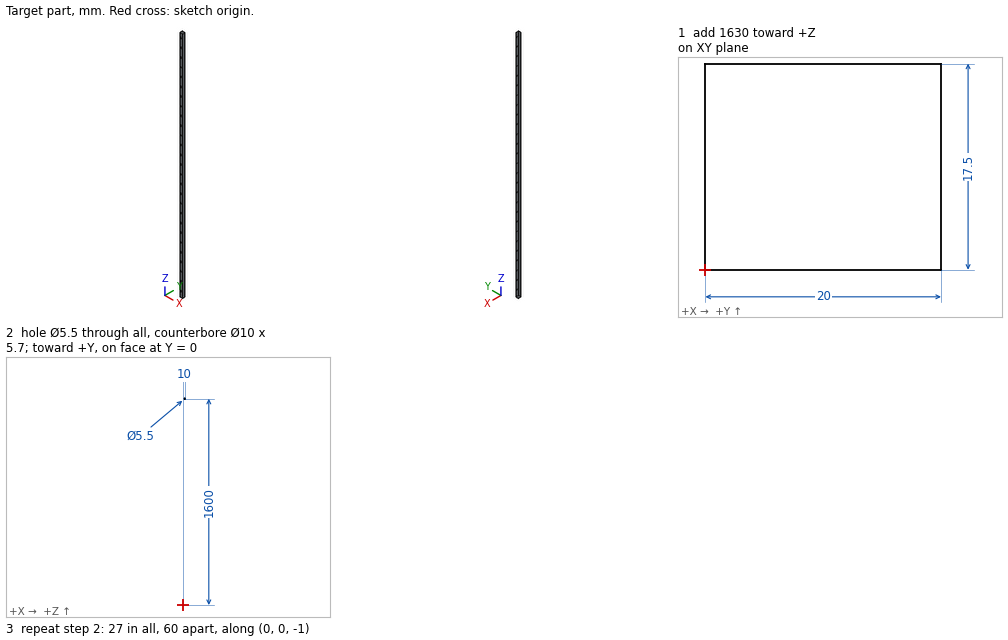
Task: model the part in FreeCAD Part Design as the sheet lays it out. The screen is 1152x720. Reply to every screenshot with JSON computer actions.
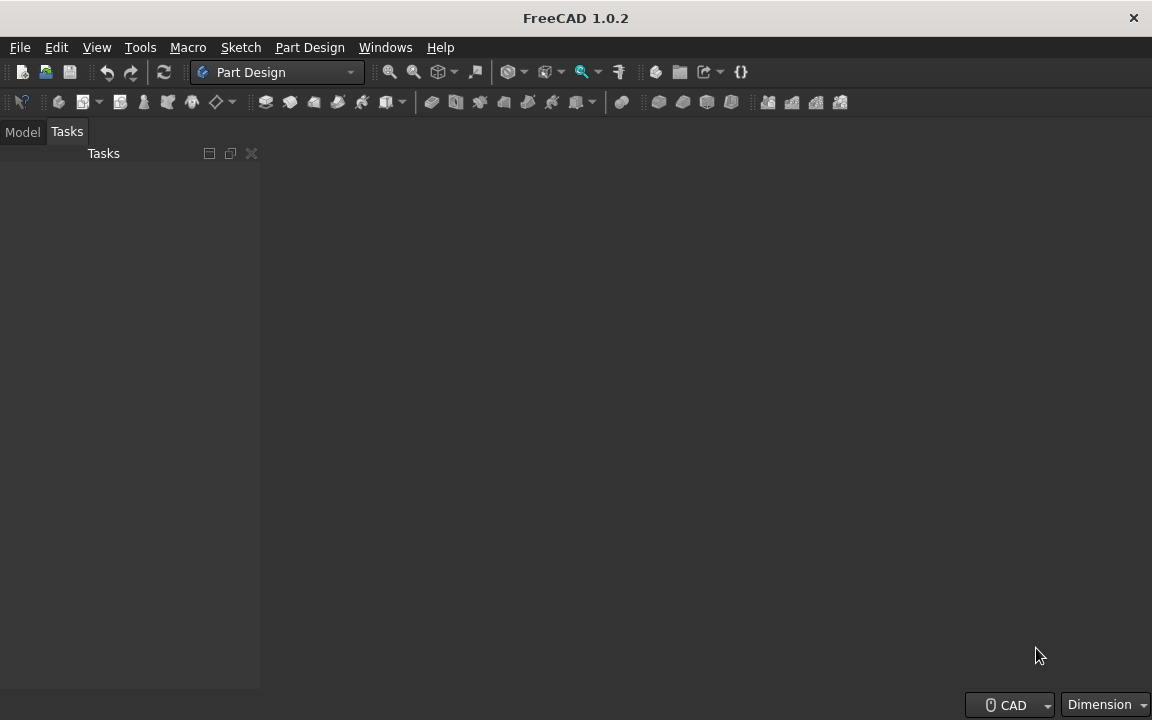
{"action": "left_click", "coordinate": [22, 72]}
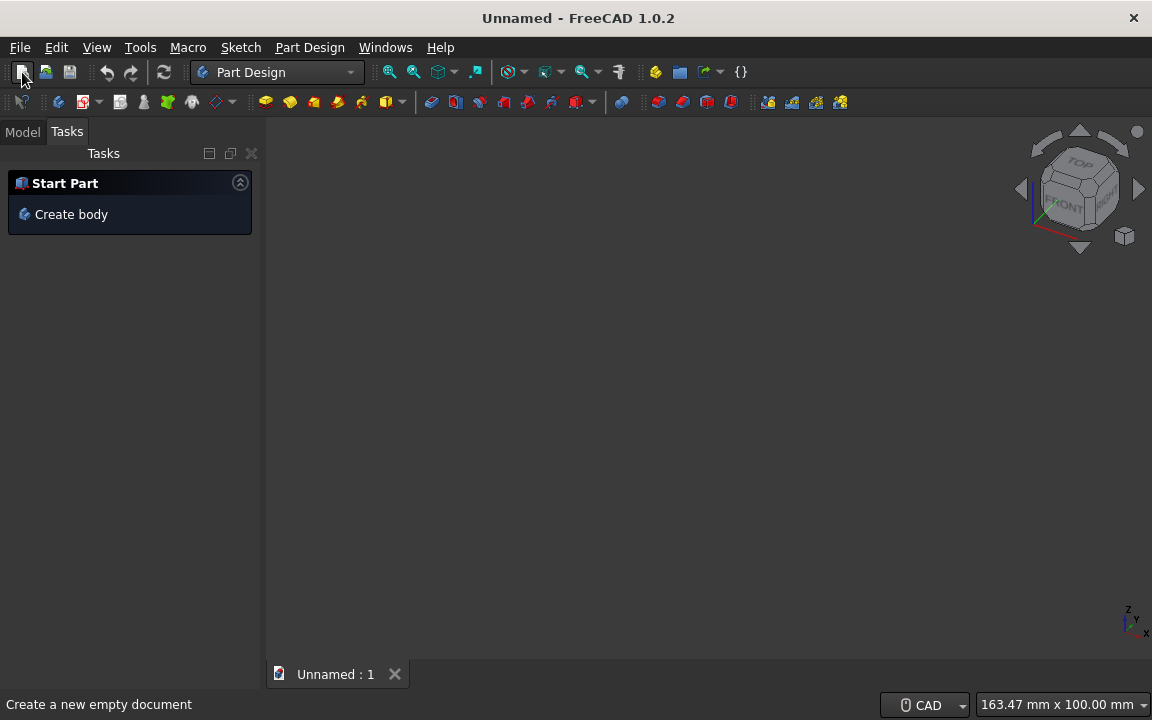
{"action": "left_click", "coordinate": [84, 102]}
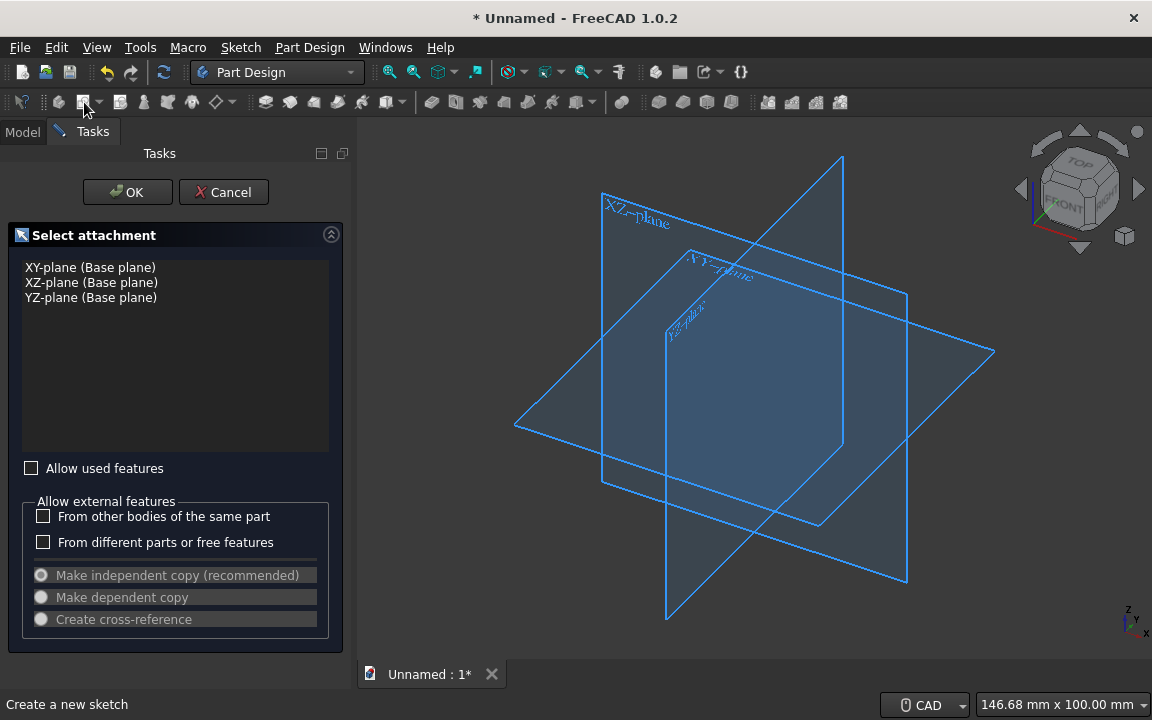
{"action": "left_click", "coordinate": [82, 268]}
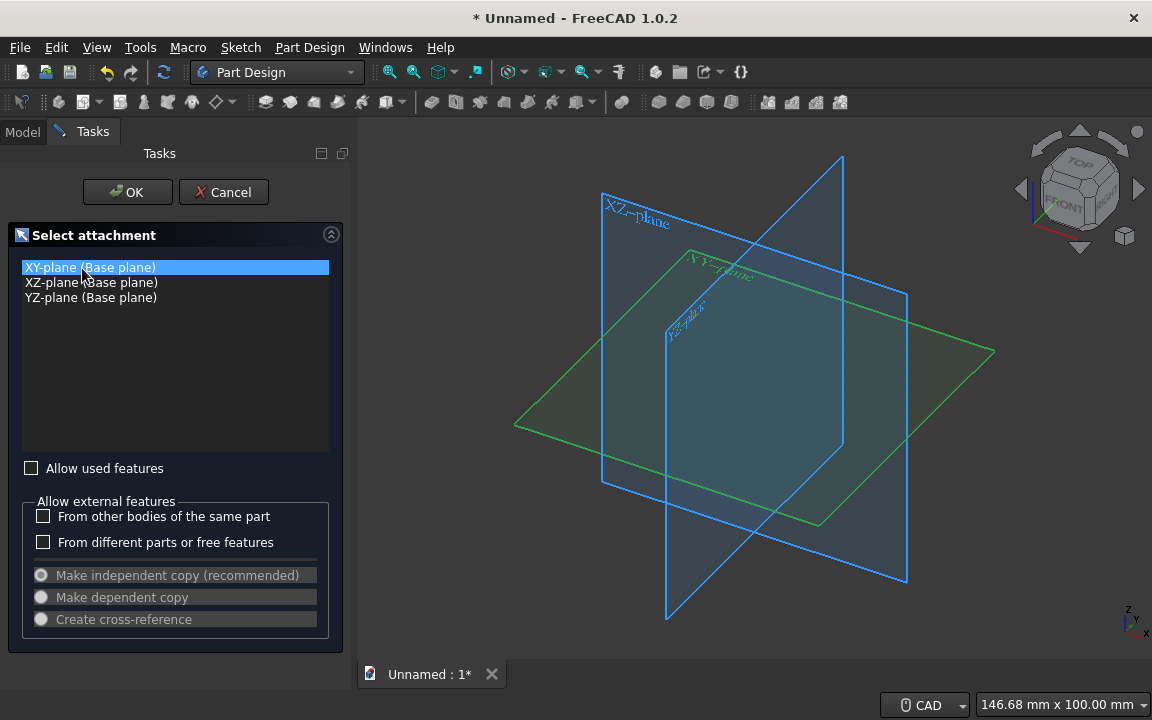
{"action": "left_click", "coordinate": [128, 192]}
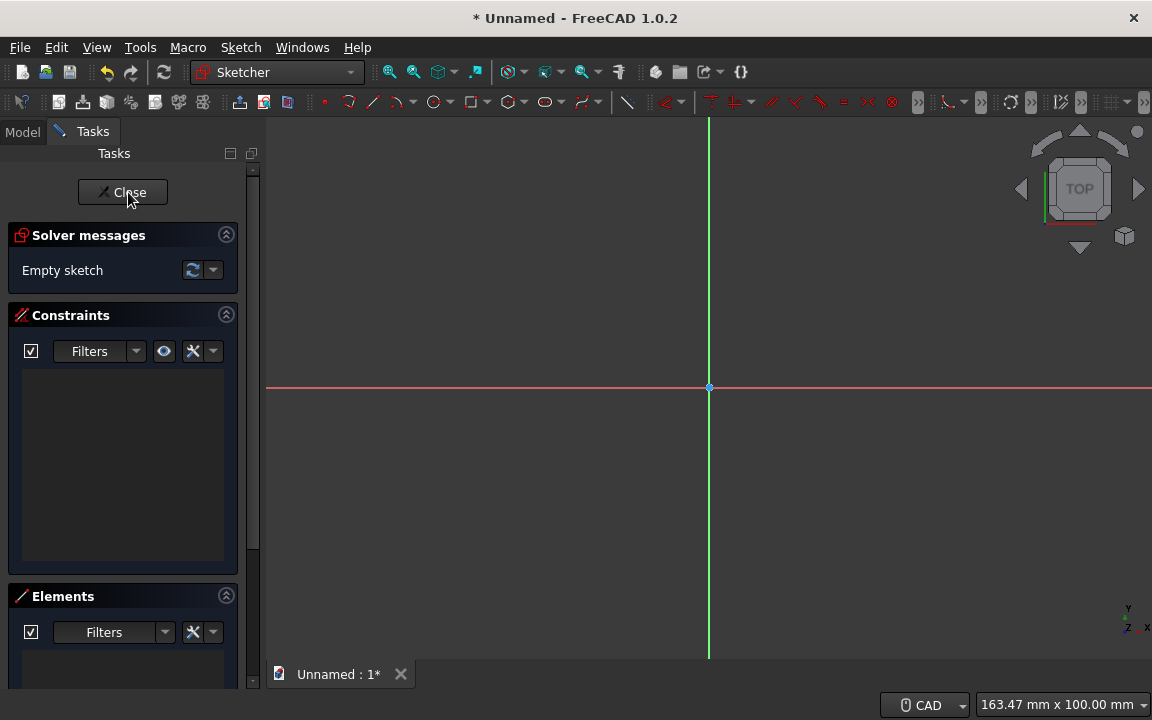
{"action": "scroll", "coordinate": [816, 320], "scroll_direction": "up", "scroll_amount": 6}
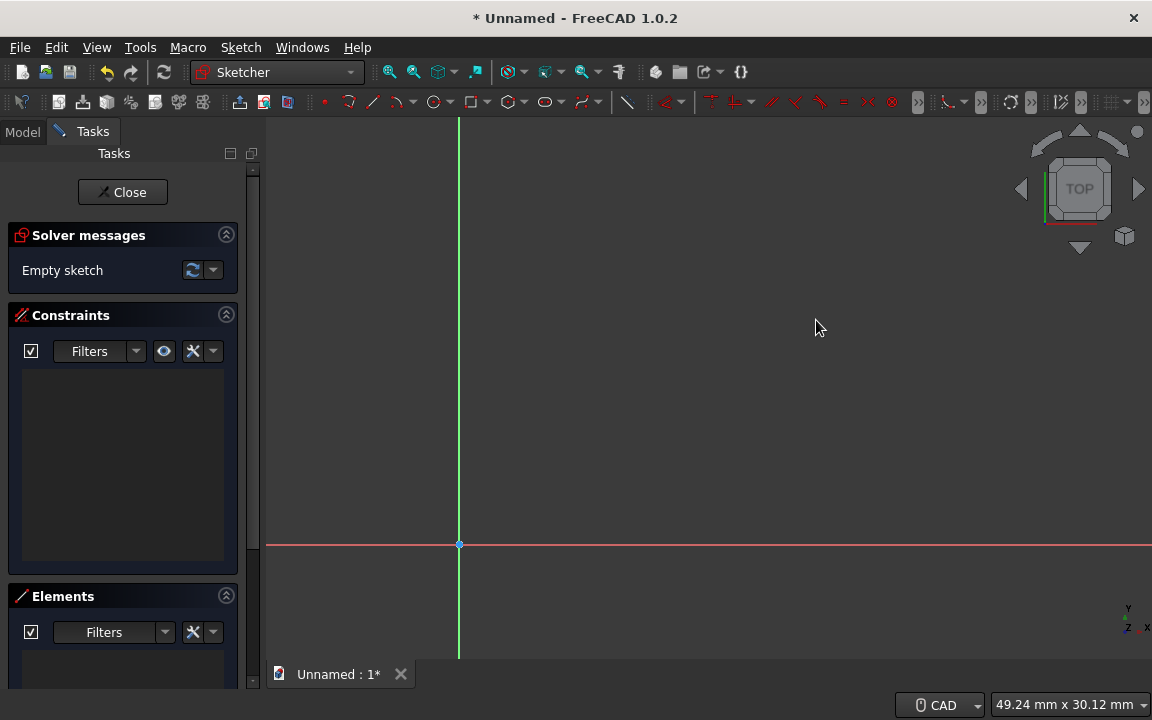
{"action": "left_click", "coordinate": [472, 102]}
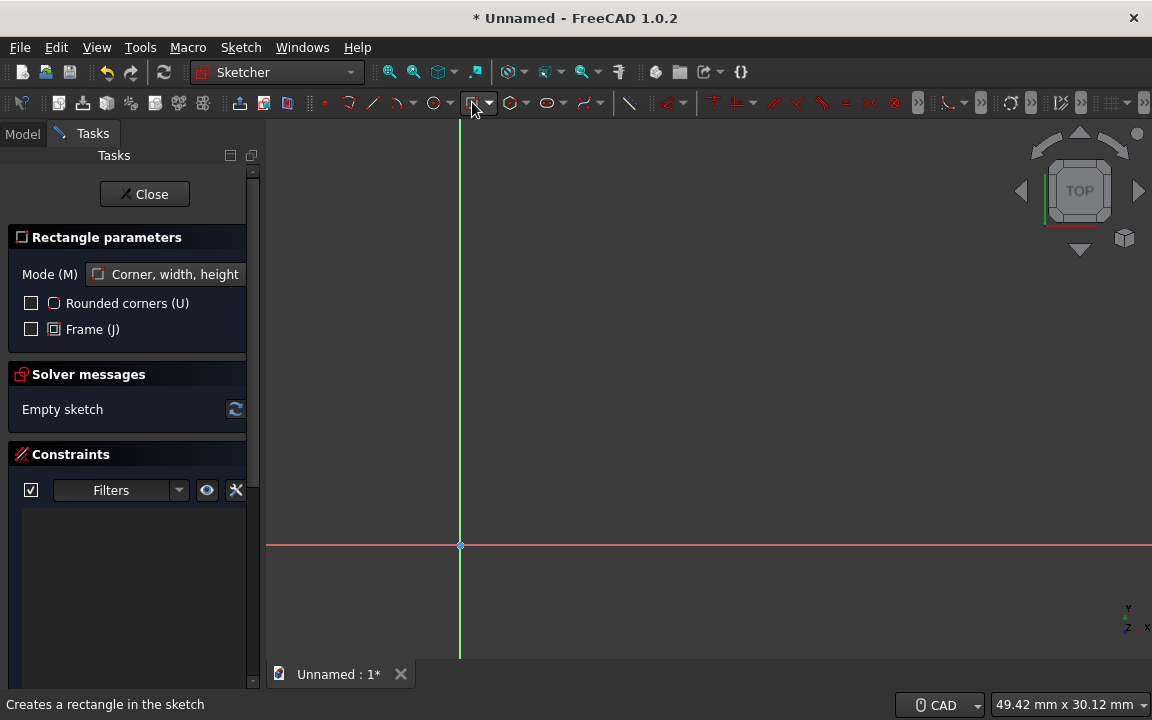
{"action": "left_click", "coordinate": [460, 545]}
{"action": "mouse_move", "coordinate": [819, 232]}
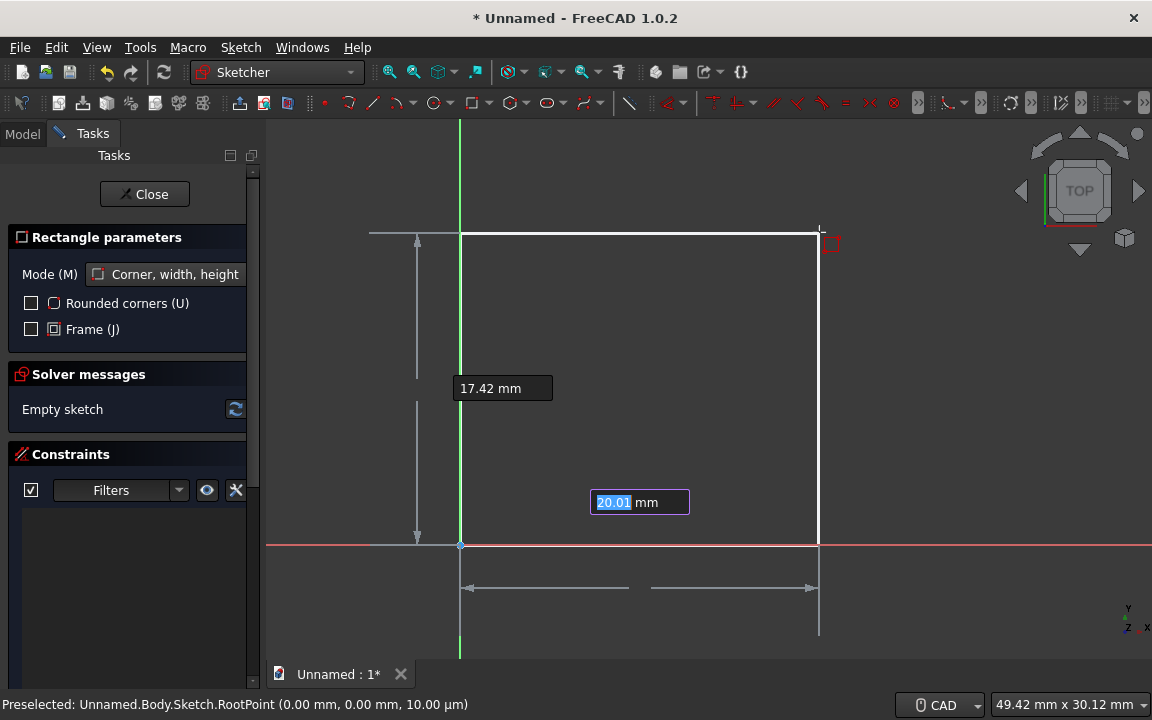
{"action": "type", "text": "20"}
{"action": "key", "text": "Tab"}
{"action": "type", "text": "17.5"}
{"action": "key", "text": "Return"}
{"action": "key", "text": "Escape"}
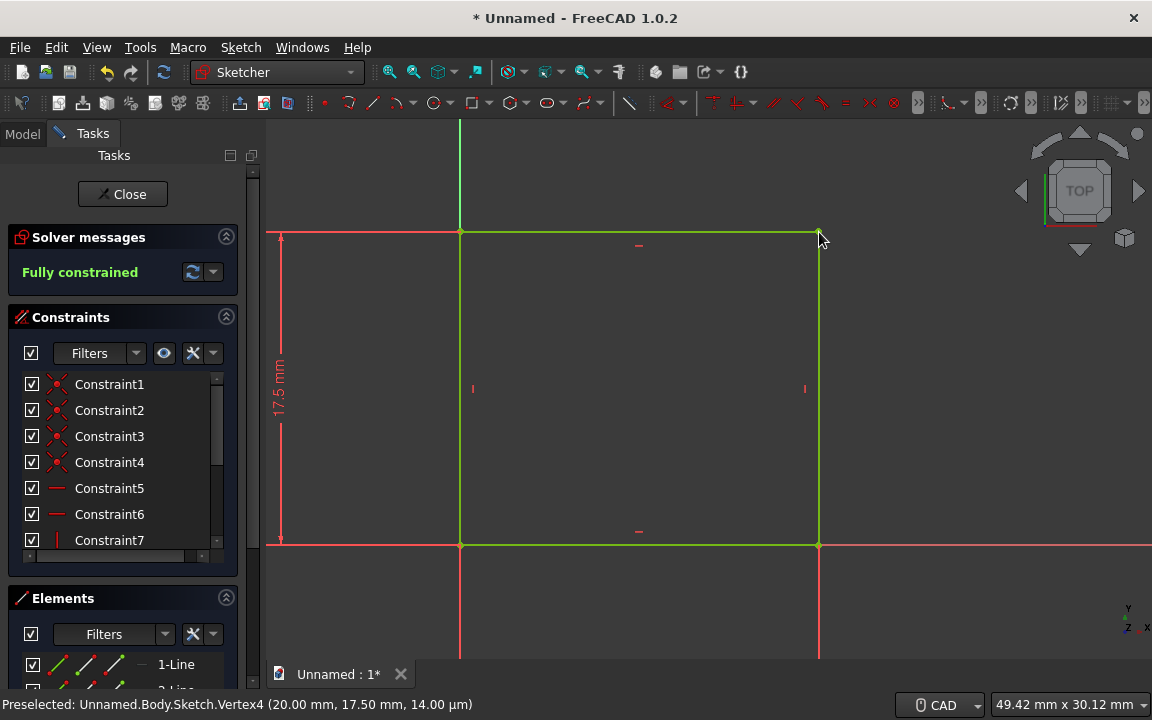
{"action": "left_click", "coordinate": [123, 194]}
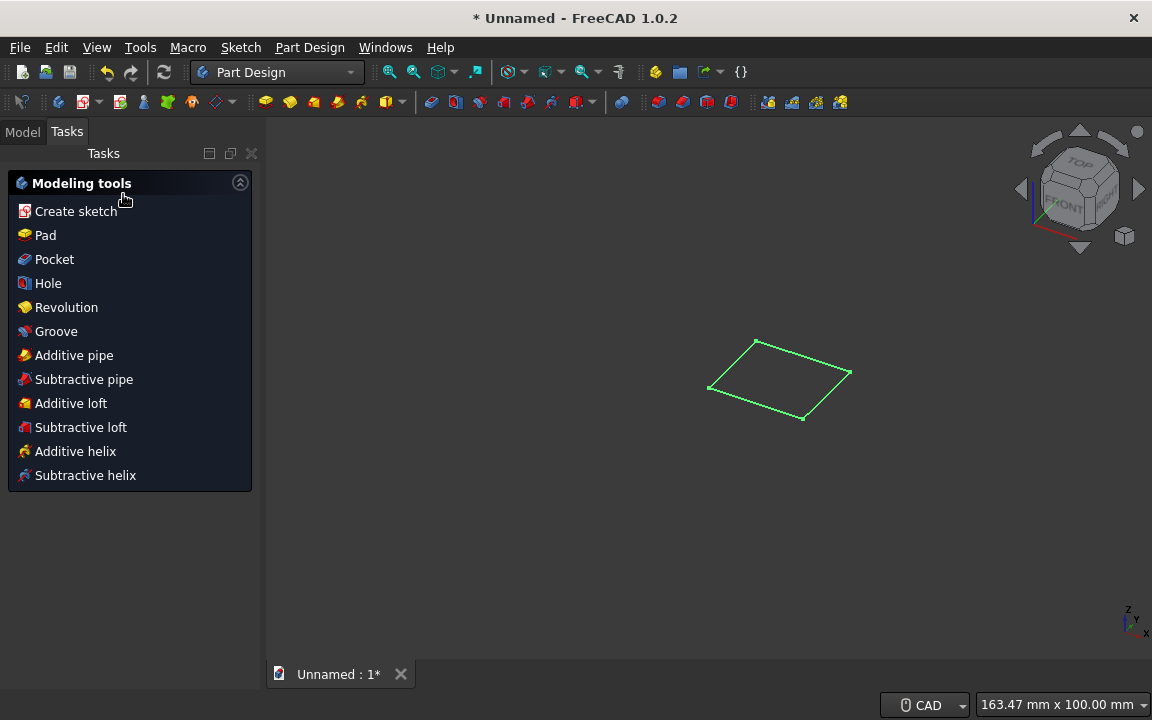
{"action": "left_click", "coordinate": [266, 102]}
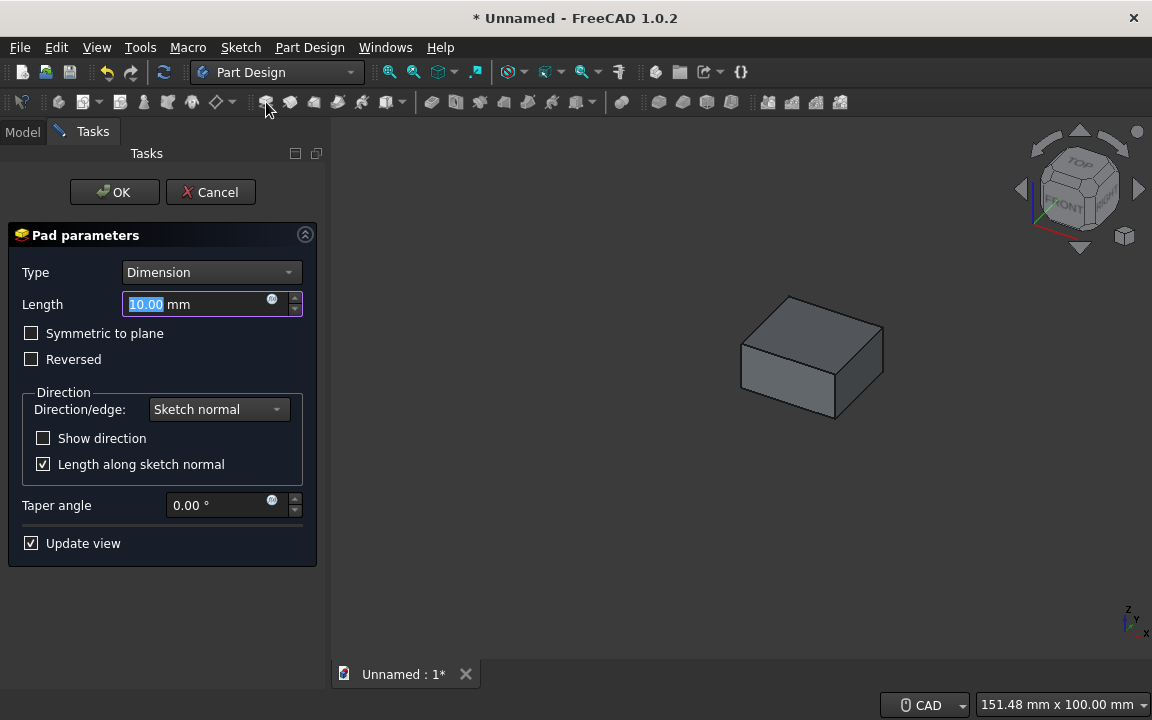
{"action": "type", "text": "1630"}
{"action": "key", "text": "Tab"}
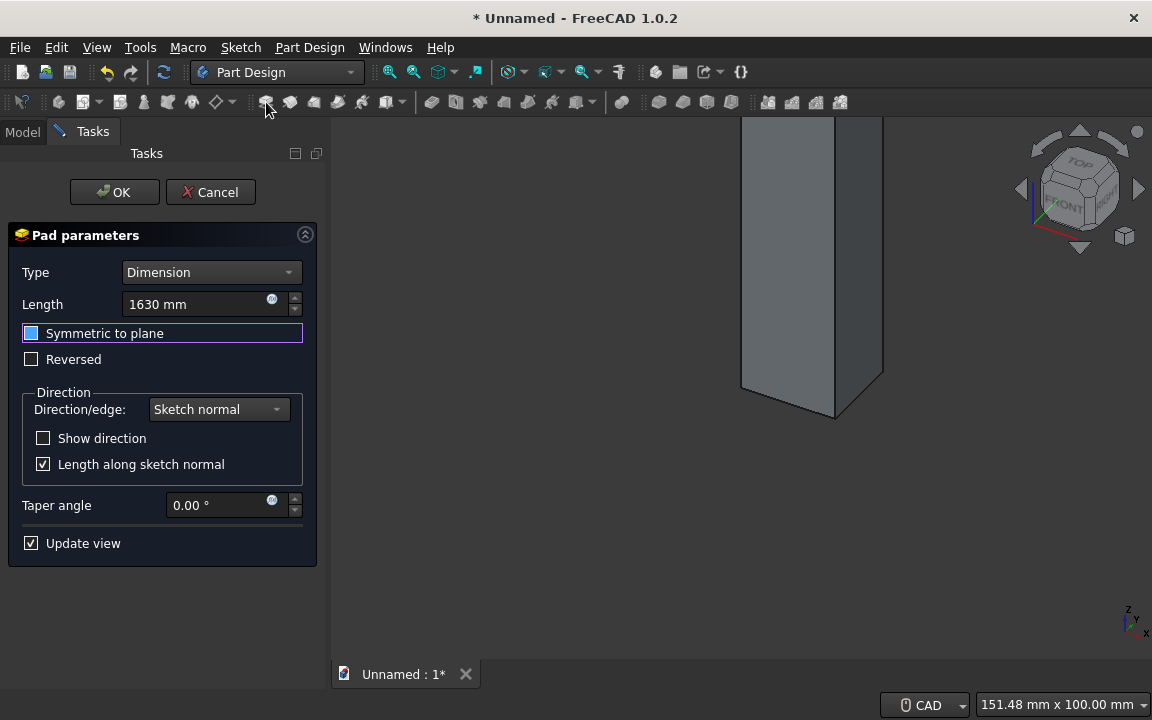
{"action": "left_click", "coordinate": [115, 192]}